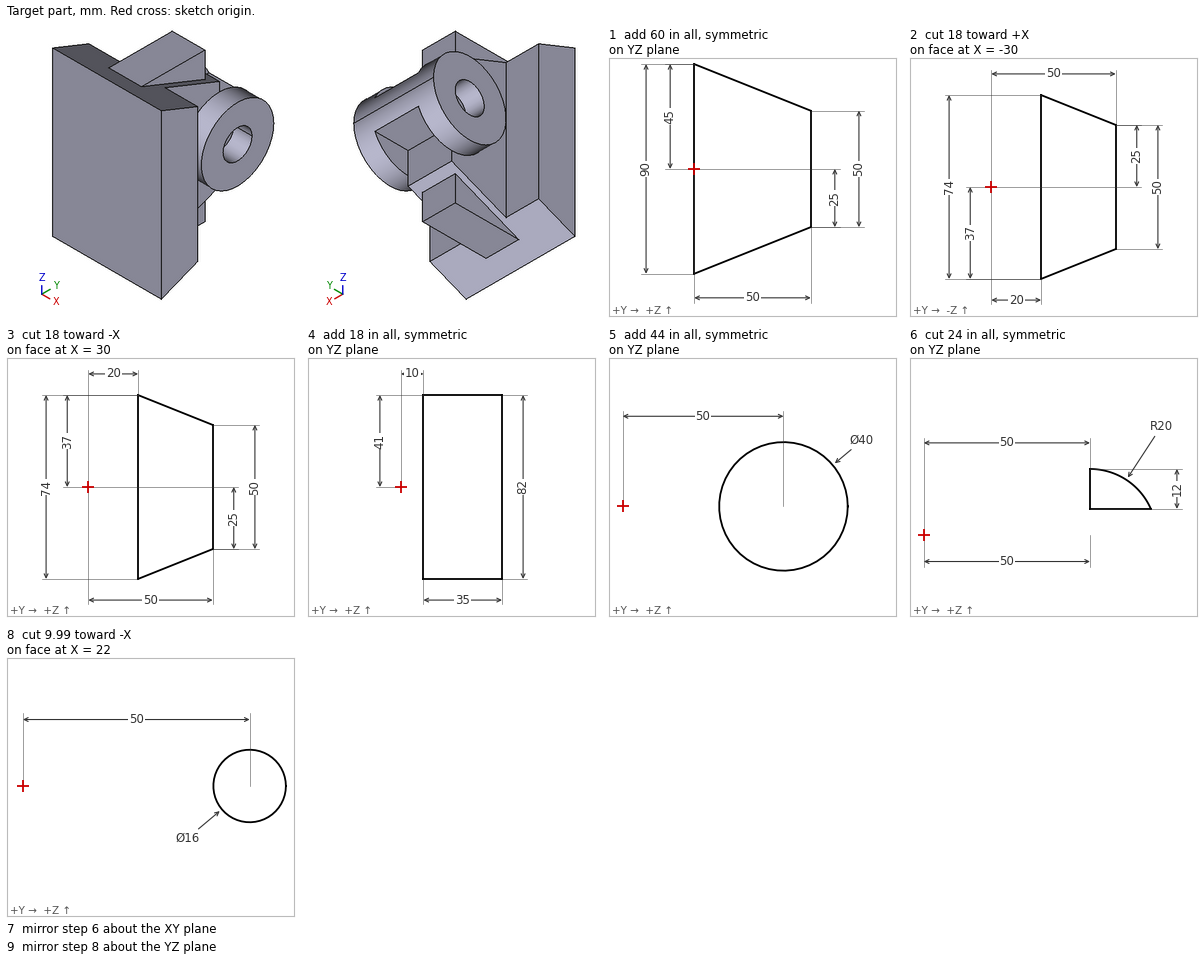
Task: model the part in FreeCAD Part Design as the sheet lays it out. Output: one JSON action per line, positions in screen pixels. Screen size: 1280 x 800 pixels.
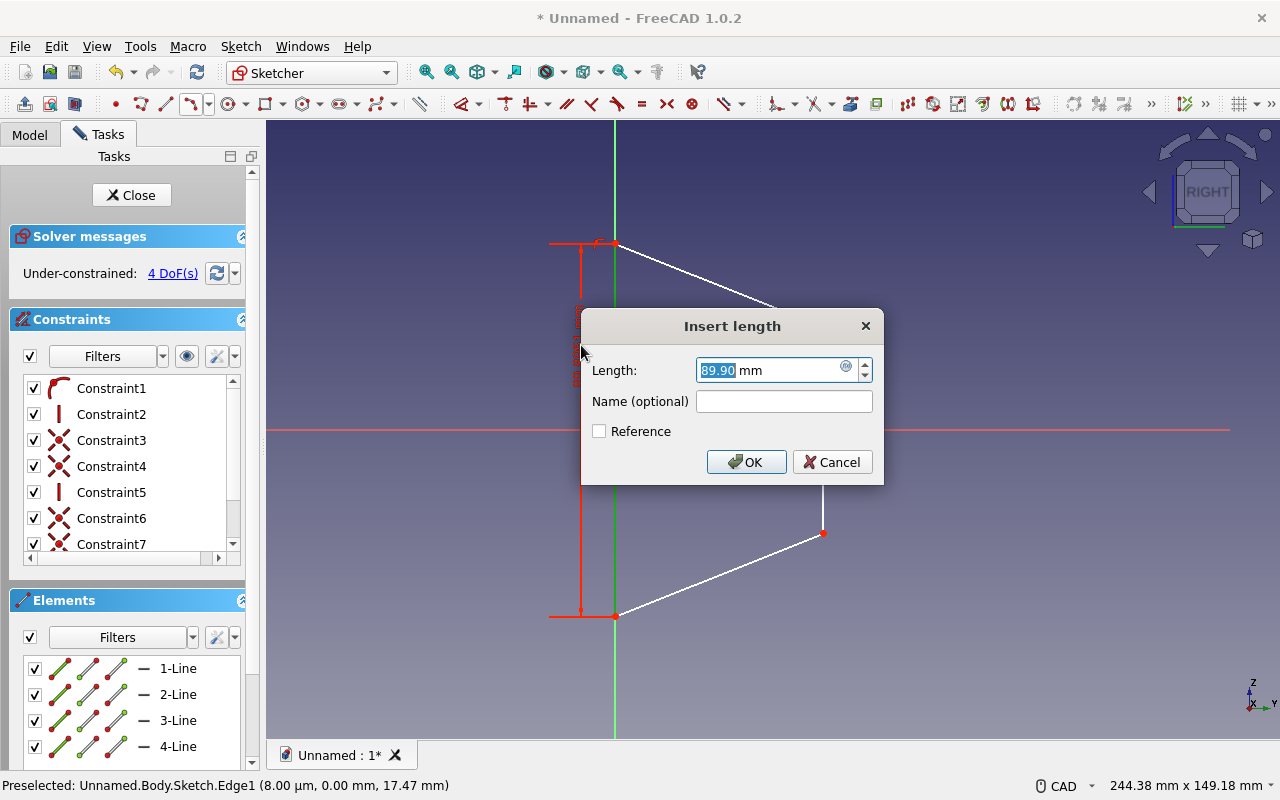
{"action": "type", "text": "90"}
{"action": "key", "text": "Return"}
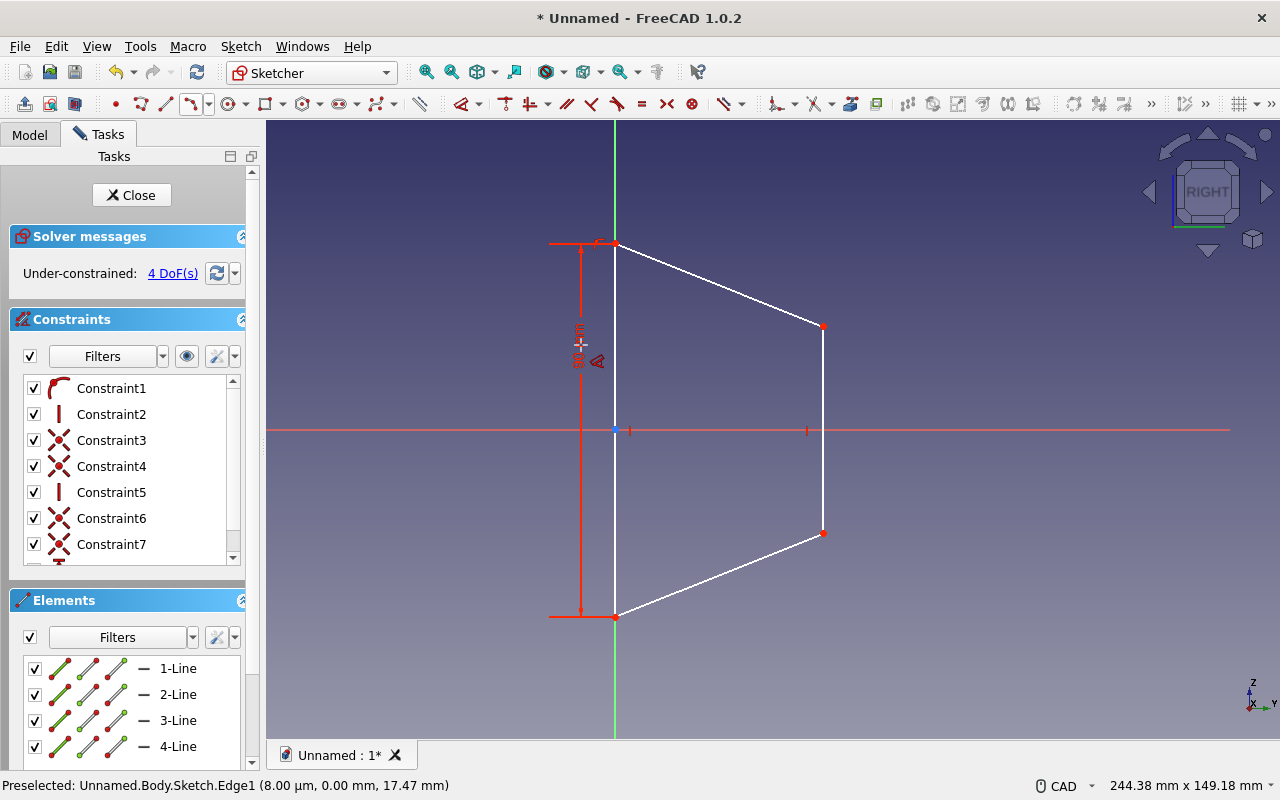
{"action": "left_click", "coordinate": [823, 472]}
{"action": "left_click", "coordinate": [857, 383]}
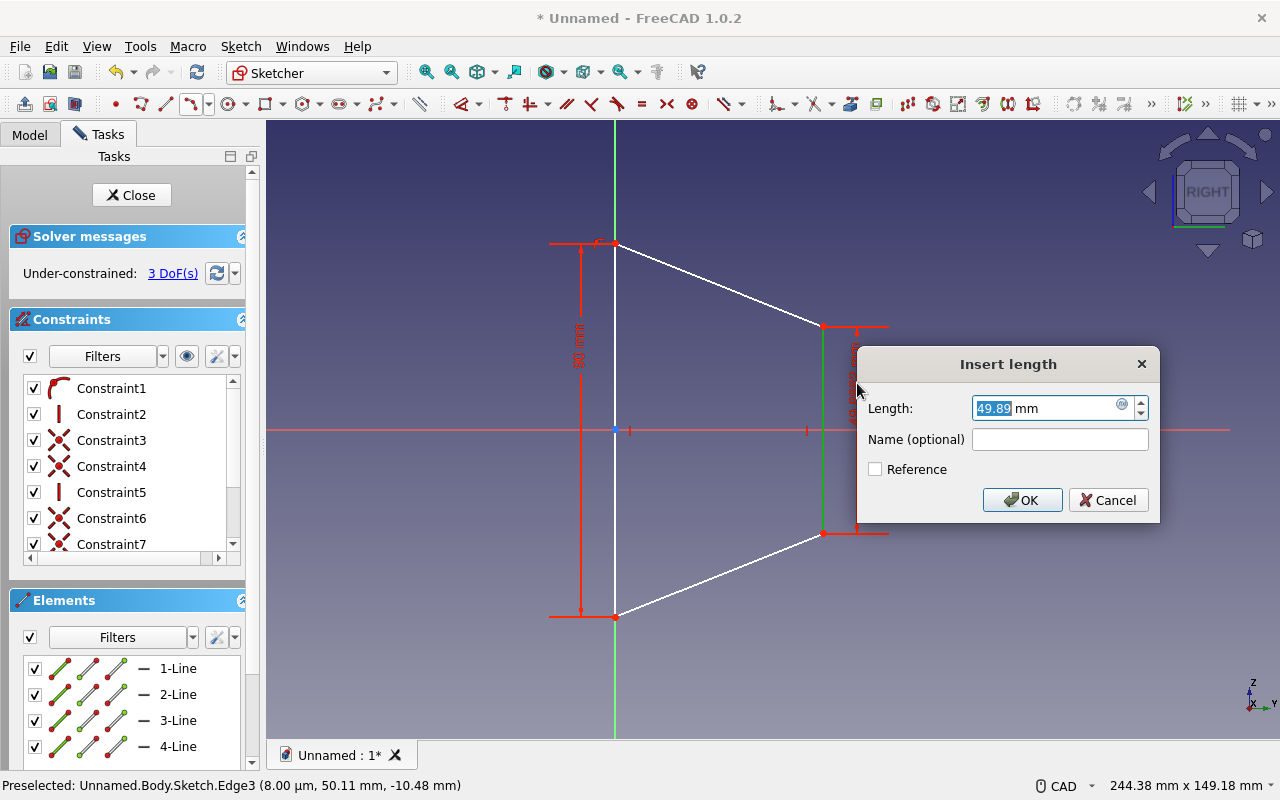
{"action": "type", "text": "50"}
{"action": "key", "text": "Return"}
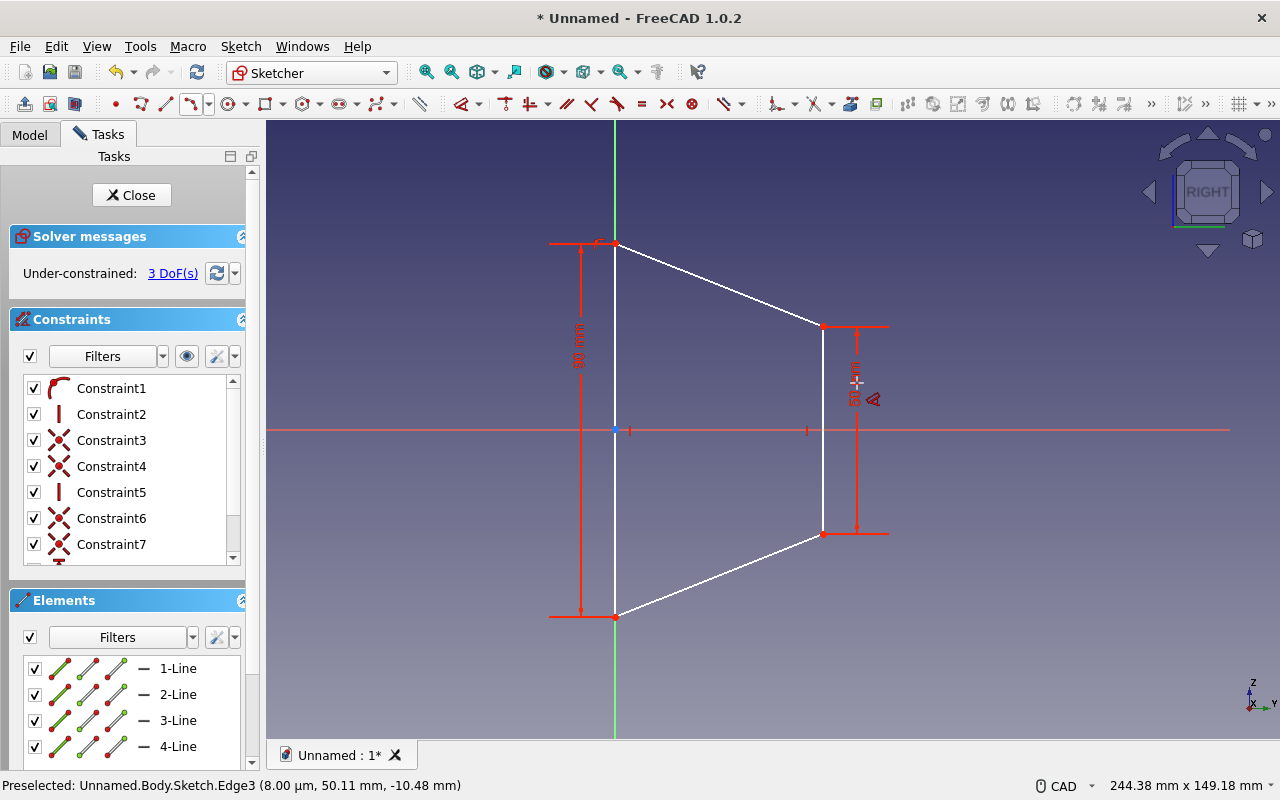
{"action": "left_click", "coordinate": [615, 244]}
{"action": "left_click", "coordinate": [581, 294]}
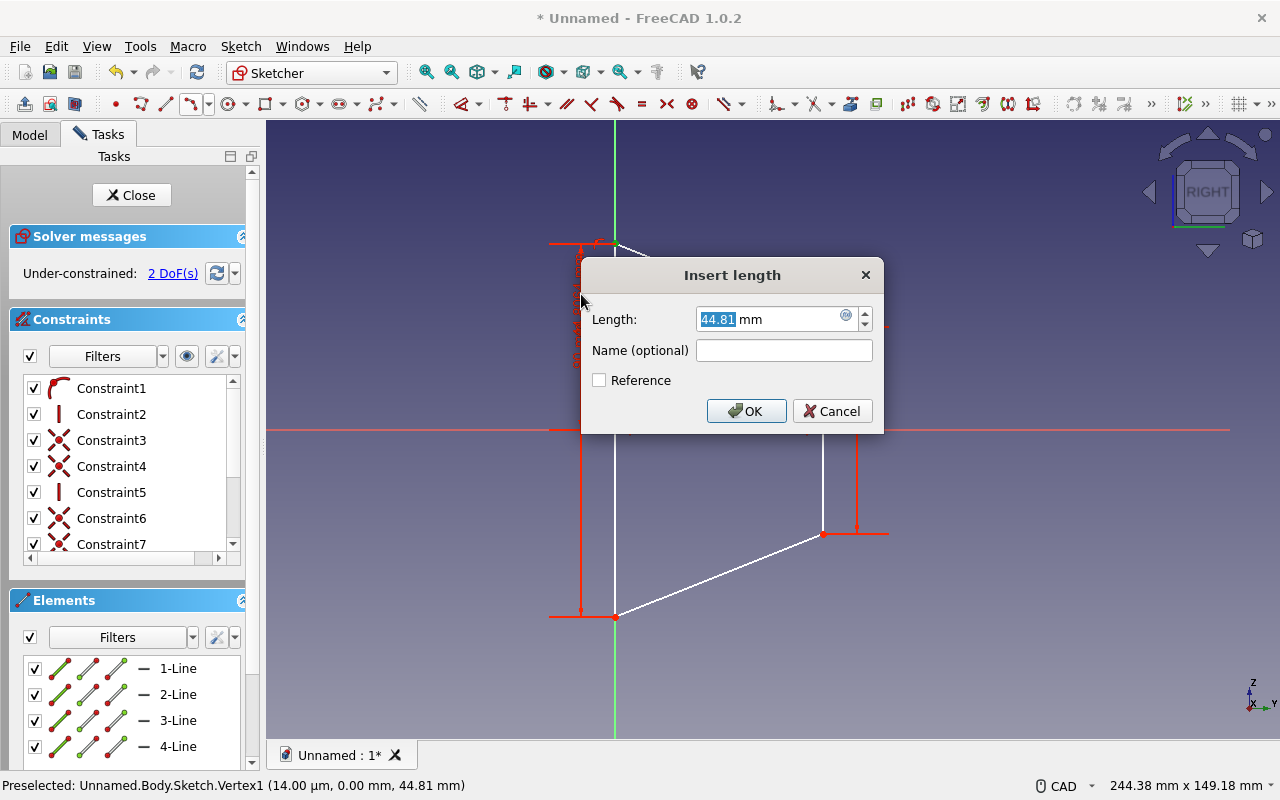
{"action": "type", "text": "45"}
{"action": "key", "text": "Return"}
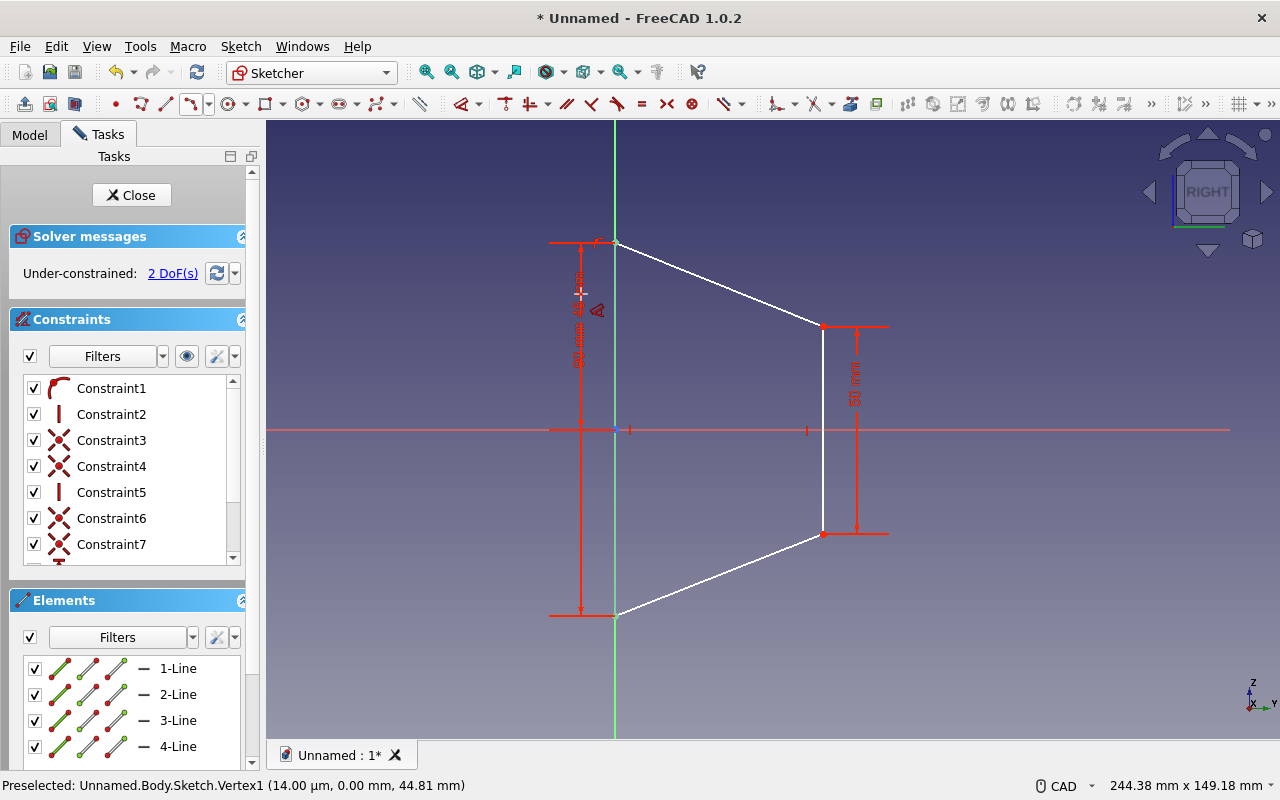
{"action": "left_click", "coordinate": [823, 534]}
{"action": "left_click", "coordinate": [671, 568]}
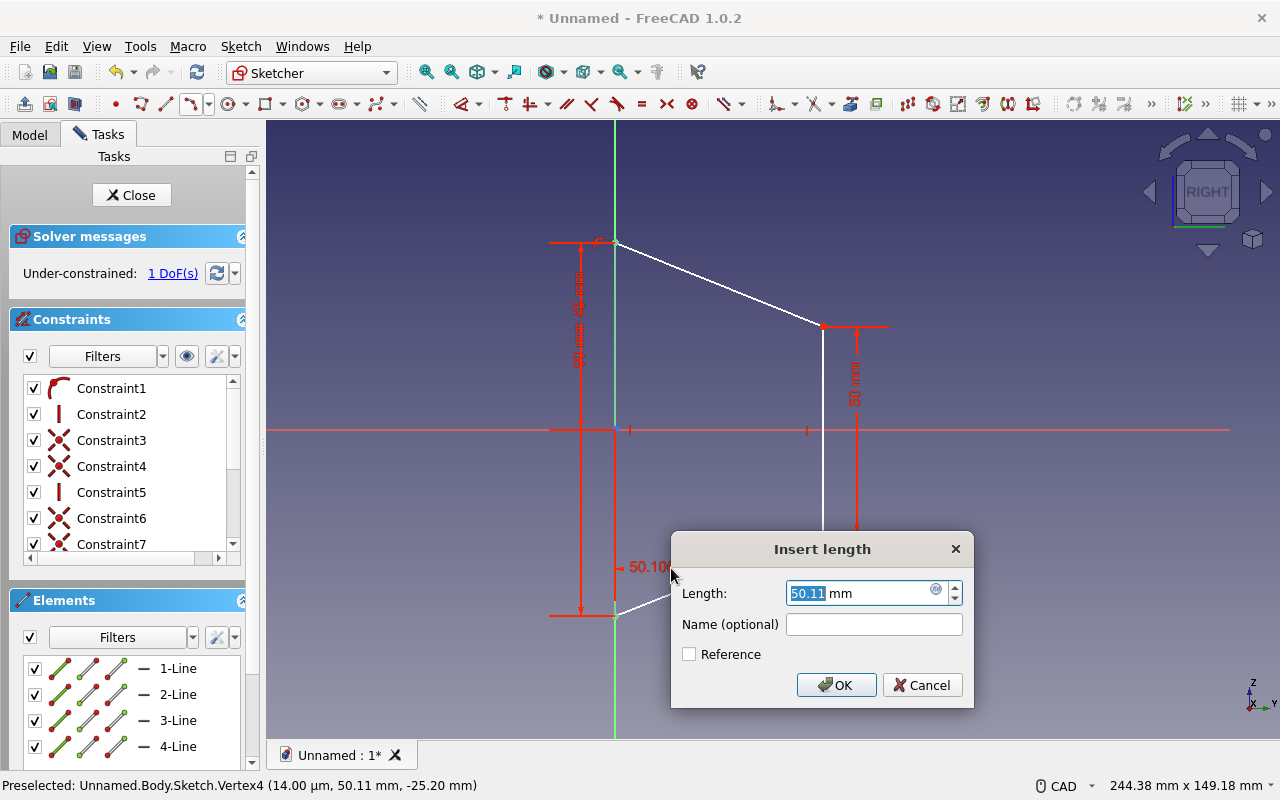
{"action": "type", "text": "50"}
{"action": "key", "text": "Return"}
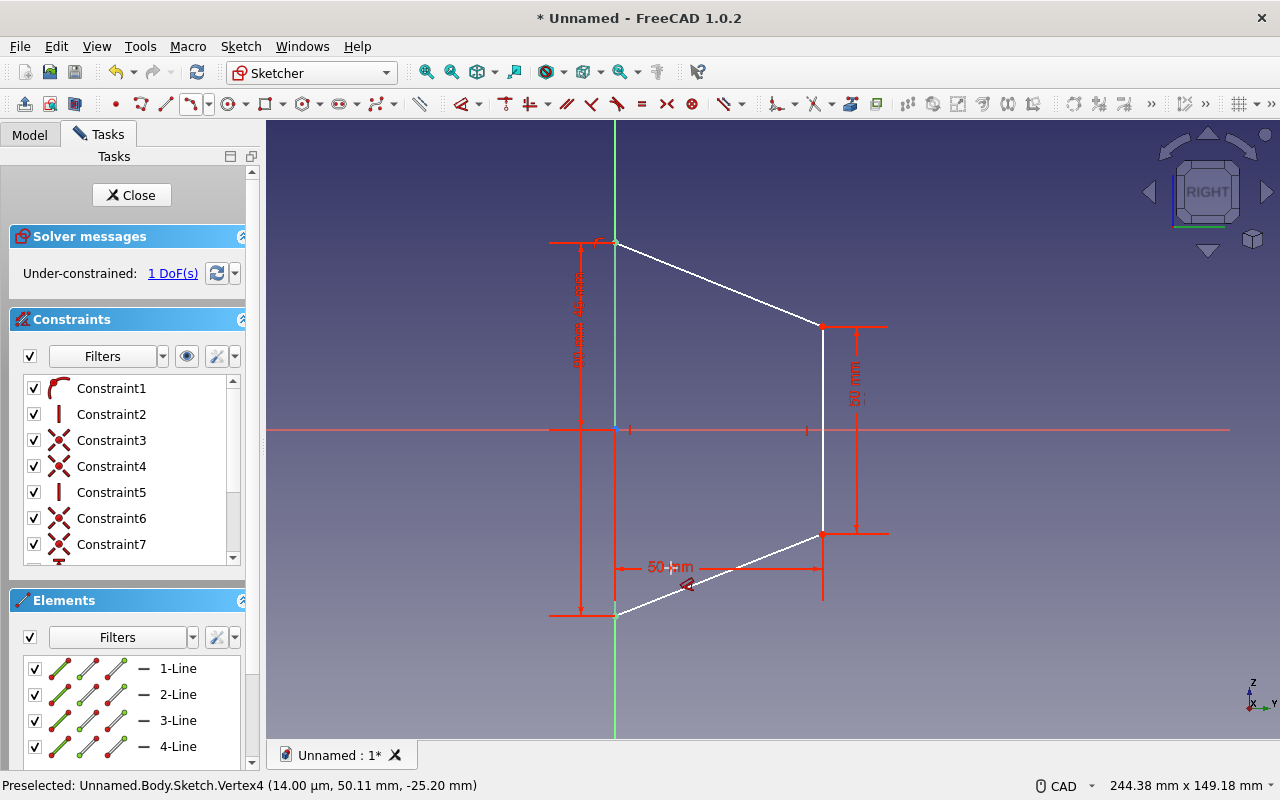
{"action": "left_click", "coordinate": [823, 534]}
{"action": "left_click", "coordinate": [857, 482]}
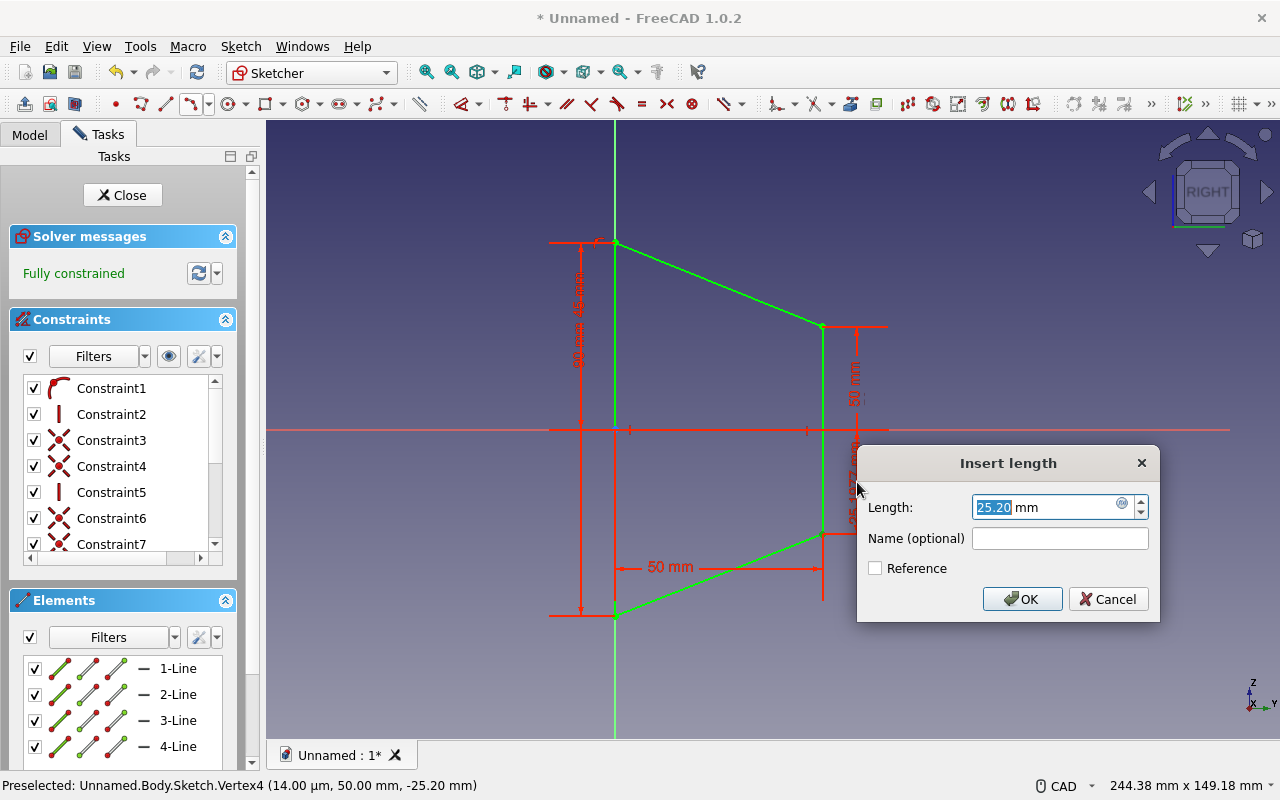
{"action": "type", "text": "25"}
{"action": "key", "text": "Return"}
{"action": "key", "text": "Escape"}